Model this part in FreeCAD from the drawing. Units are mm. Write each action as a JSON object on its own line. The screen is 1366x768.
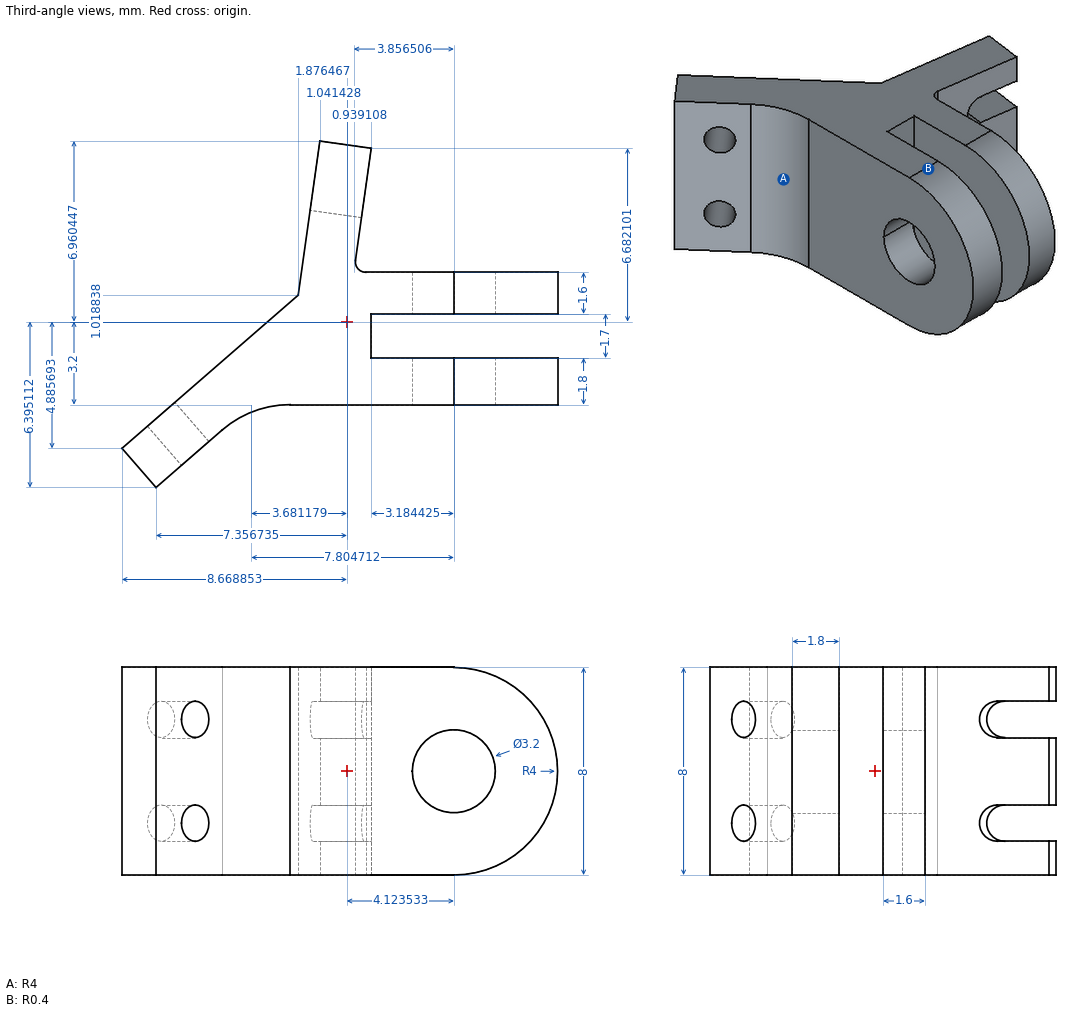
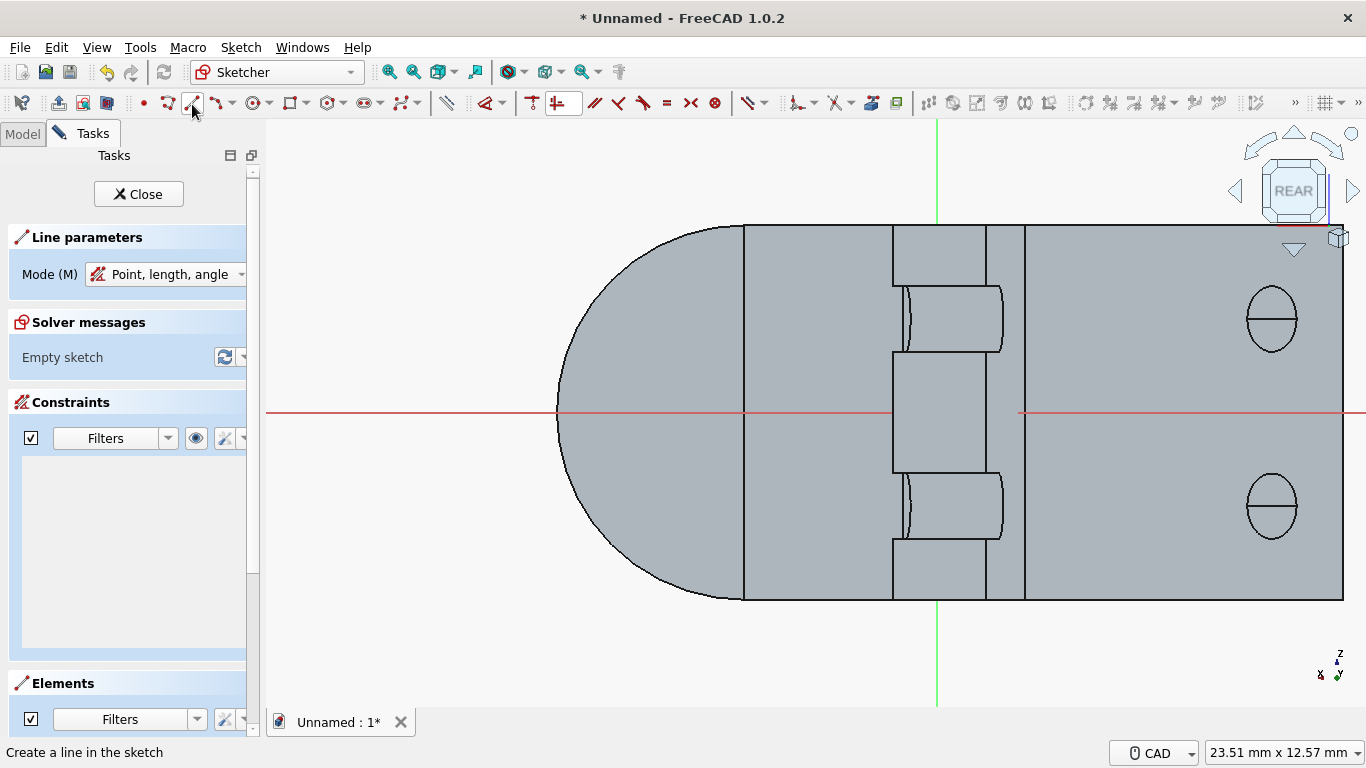
{"action": "left_click", "coordinate": [744, 600]}
{"action": "left_click", "coordinate": [744, 225]}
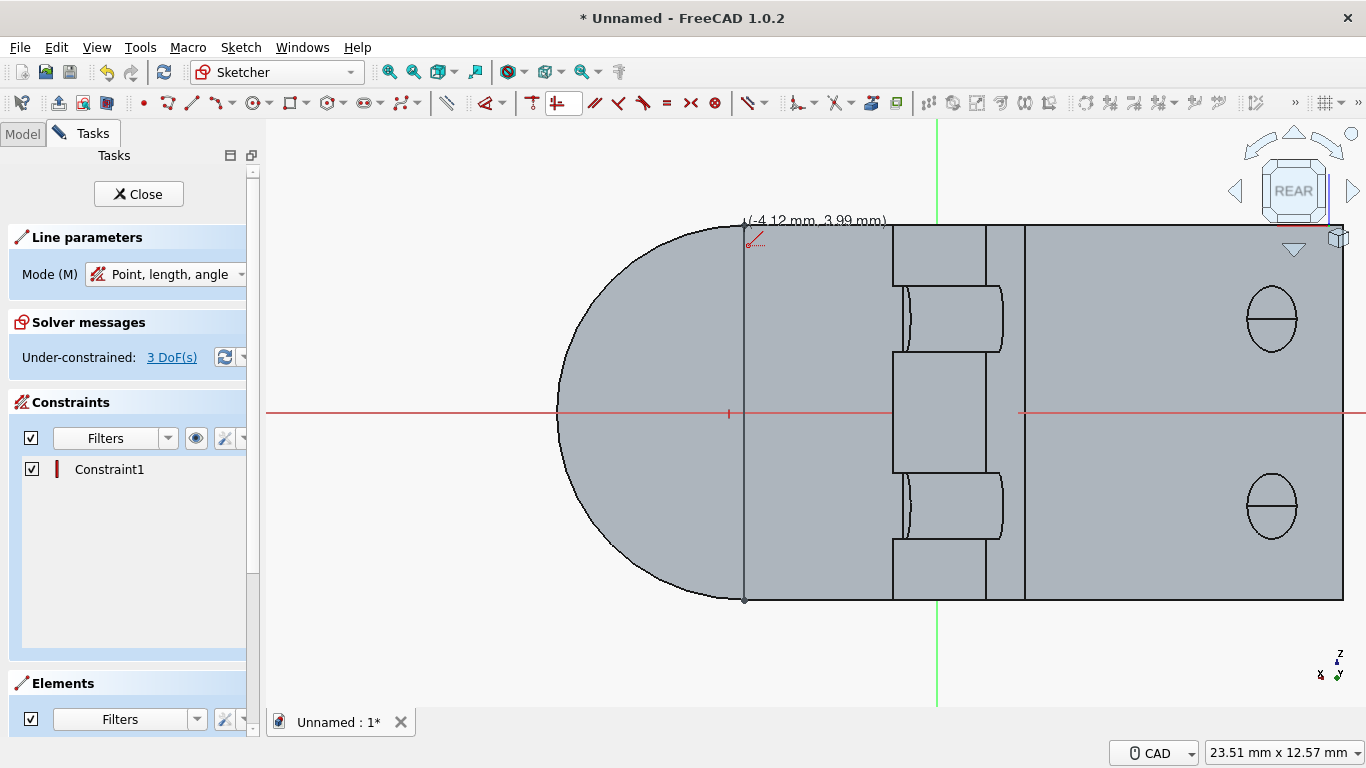
{"action": "left_click", "coordinate": [216, 104]}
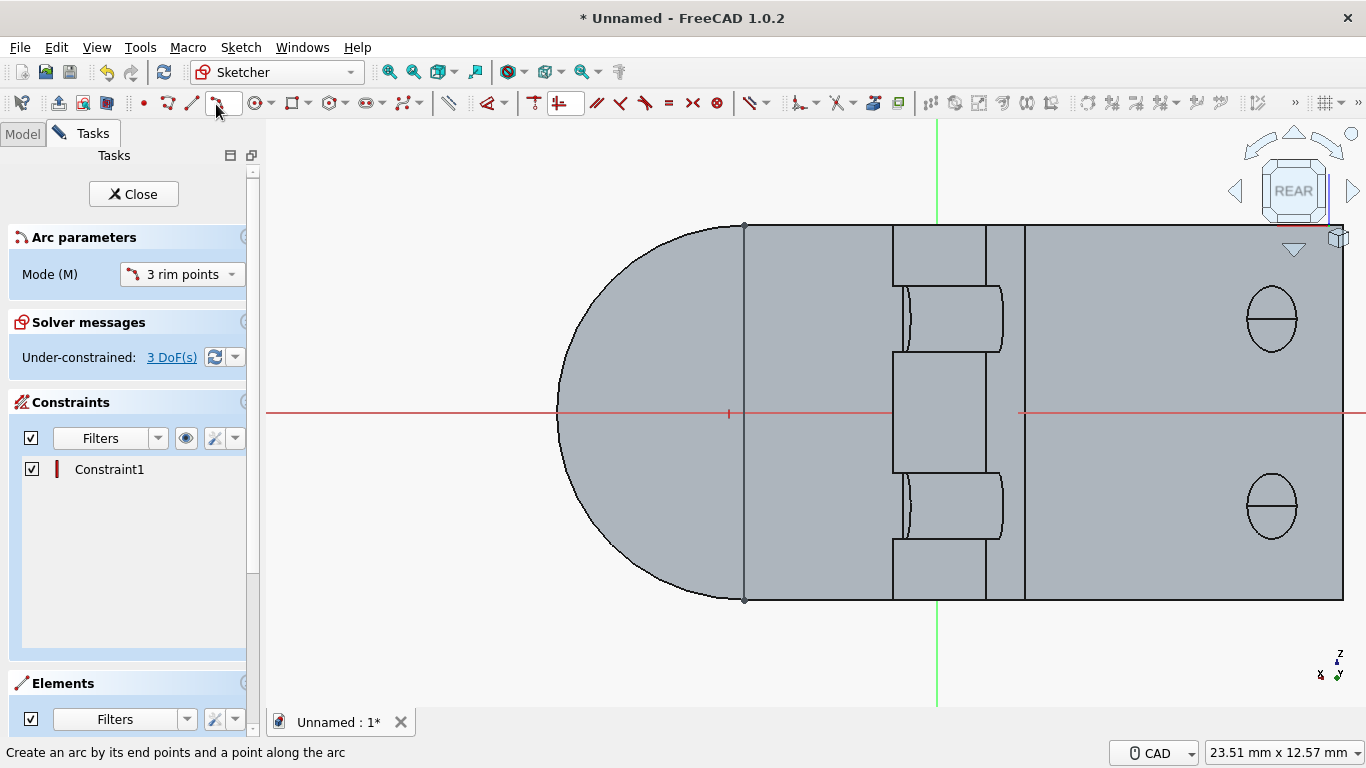
{"action": "left_click", "coordinate": [744, 226]}
{"action": "left_click", "coordinate": [744, 601]}
{"action": "left_click", "coordinate": [566, 355]}
{"action": "key", "text": "Escape"}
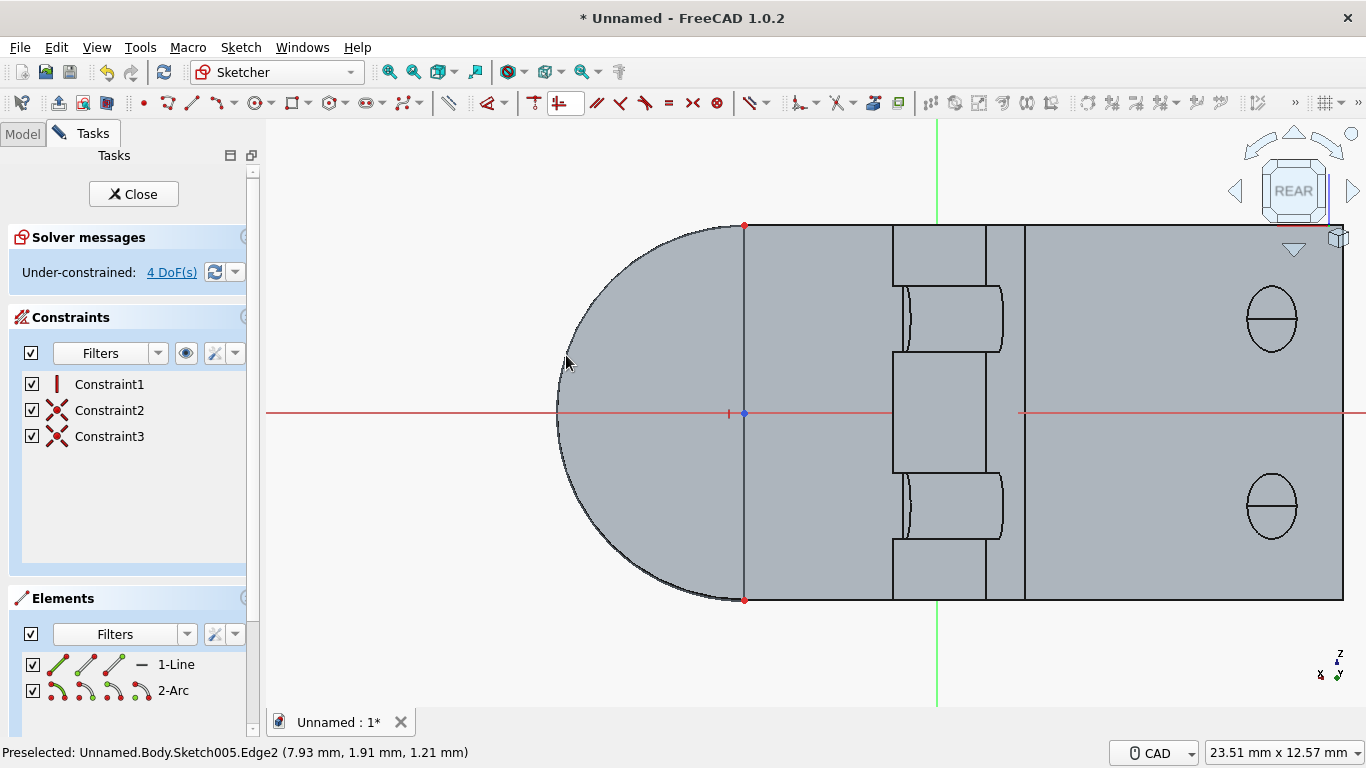
{"action": "left_click", "coordinate": [744, 414]}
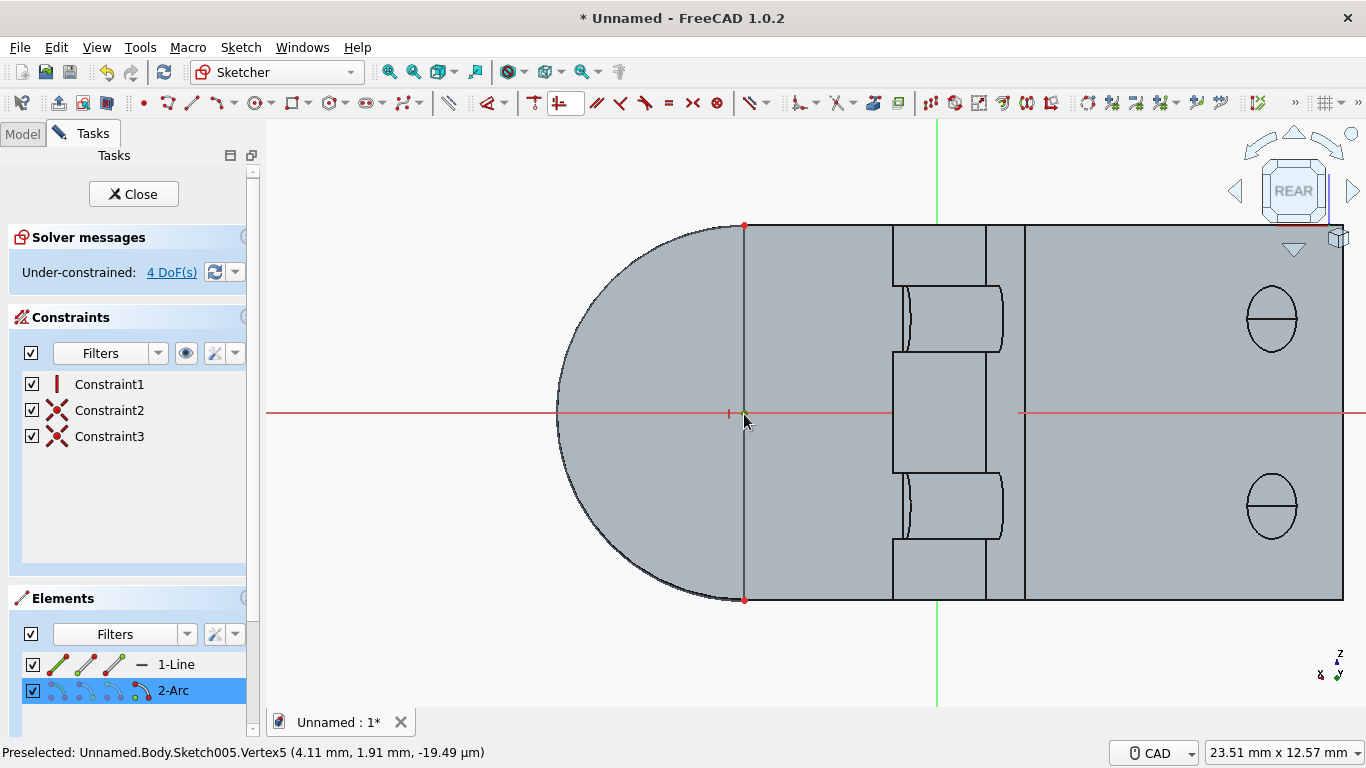
{"action": "left_click", "coordinate": [359, 413]}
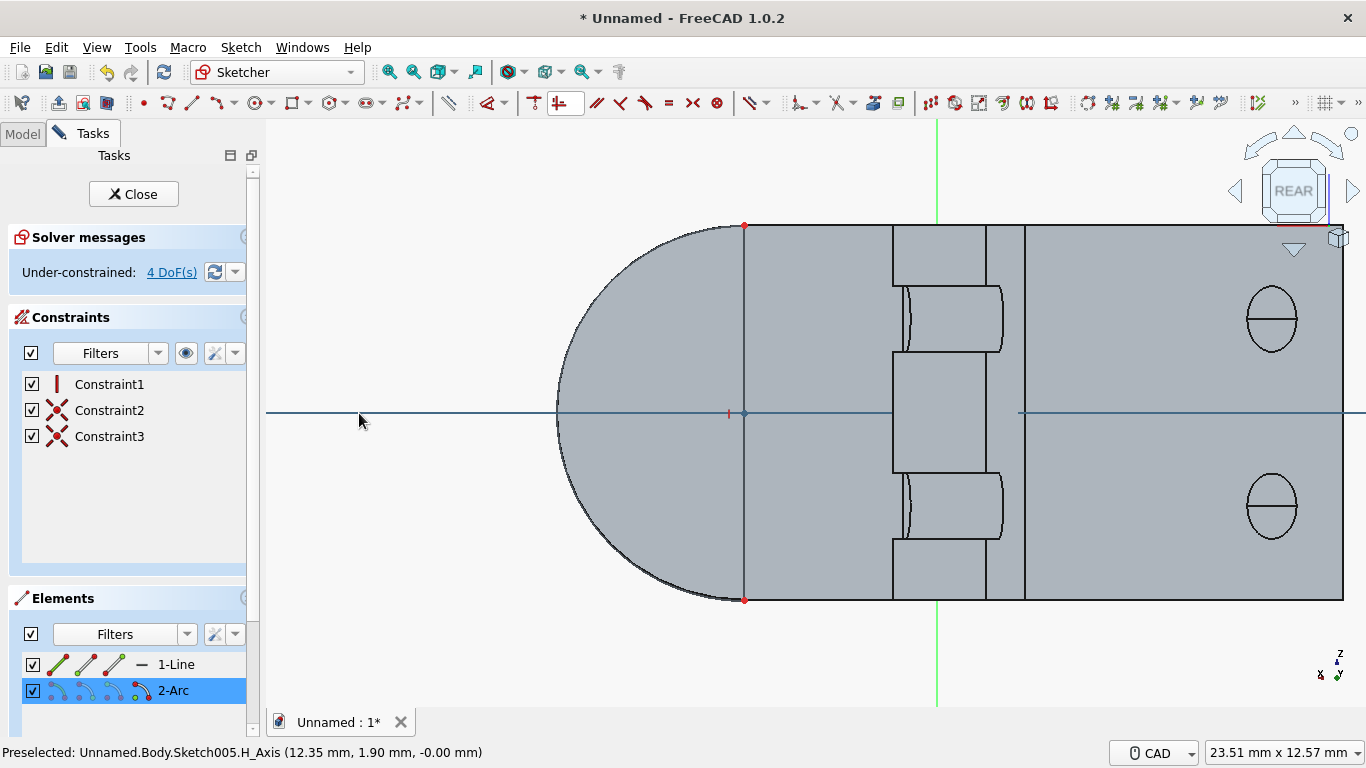
{"action": "left_click", "coordinate": [534, 104]}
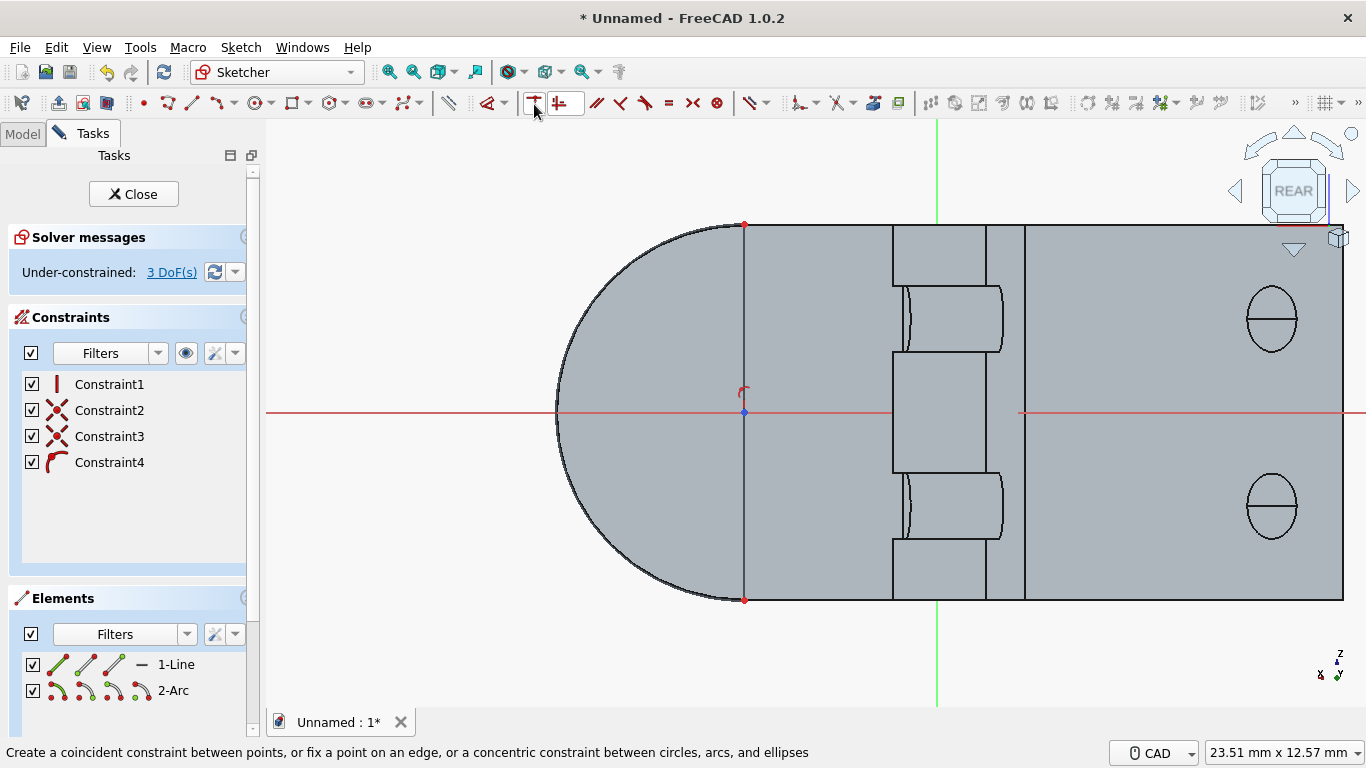
{"action": "left_click", "coordinate": [488, 104]}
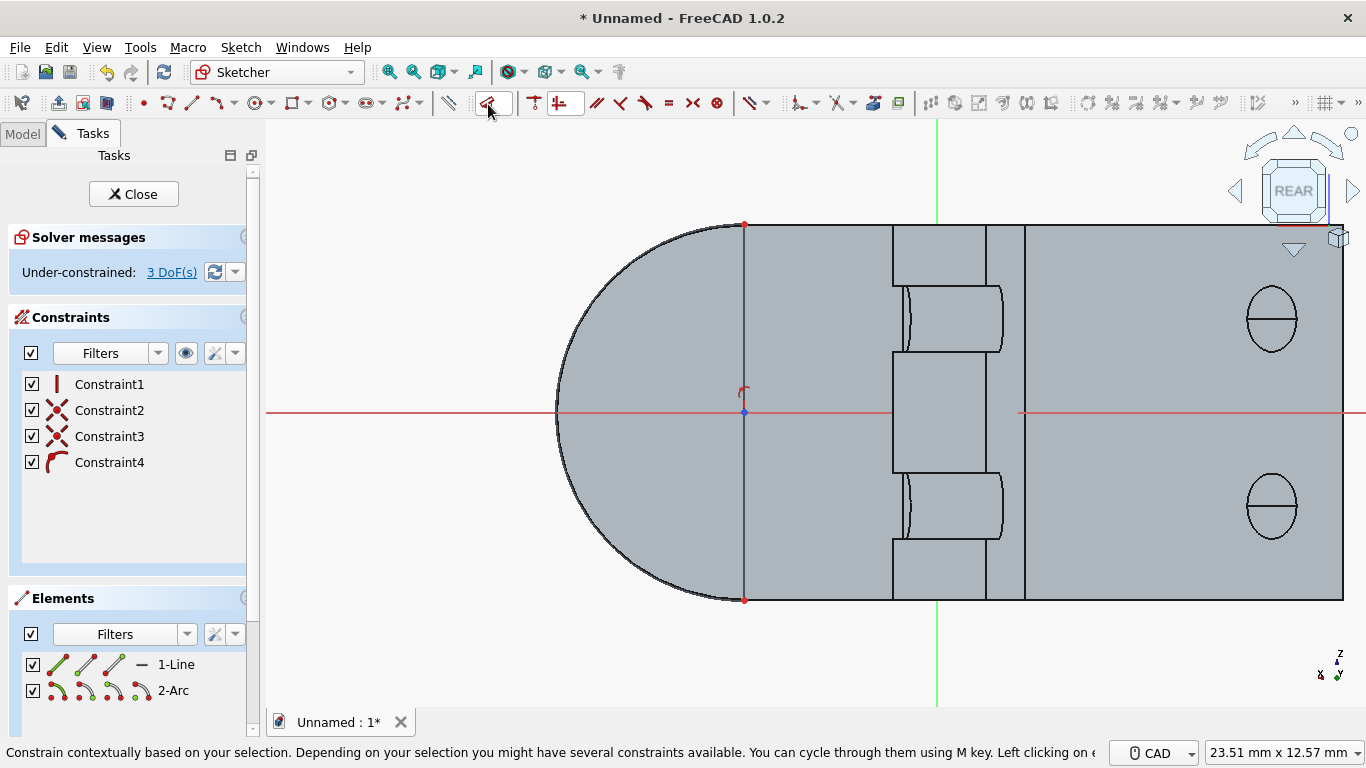
{"action": "left_click", "coordinate": [592, 302]}
{"action": "left_click", "coordinate": [566, 283]}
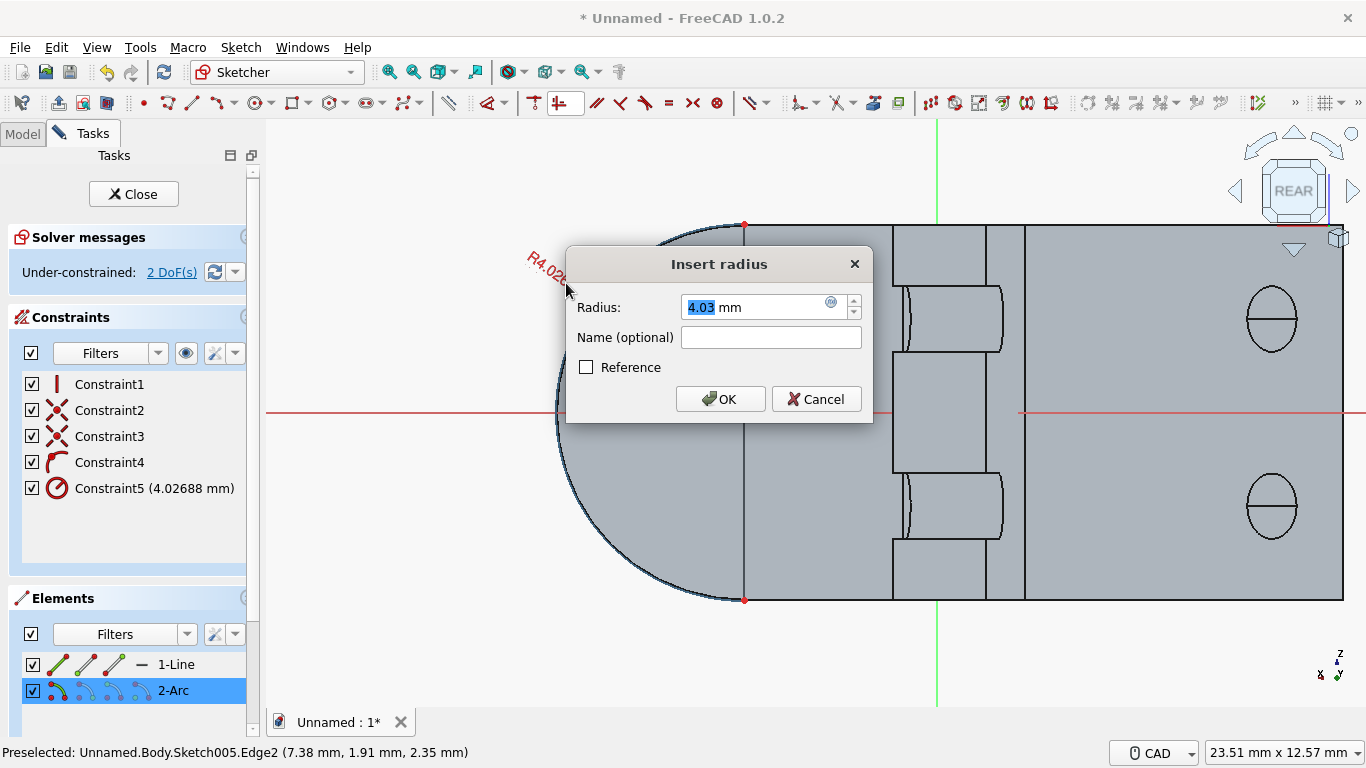
{"action": "type", "text": "4"}
{"action": "key", "text": "Return"}